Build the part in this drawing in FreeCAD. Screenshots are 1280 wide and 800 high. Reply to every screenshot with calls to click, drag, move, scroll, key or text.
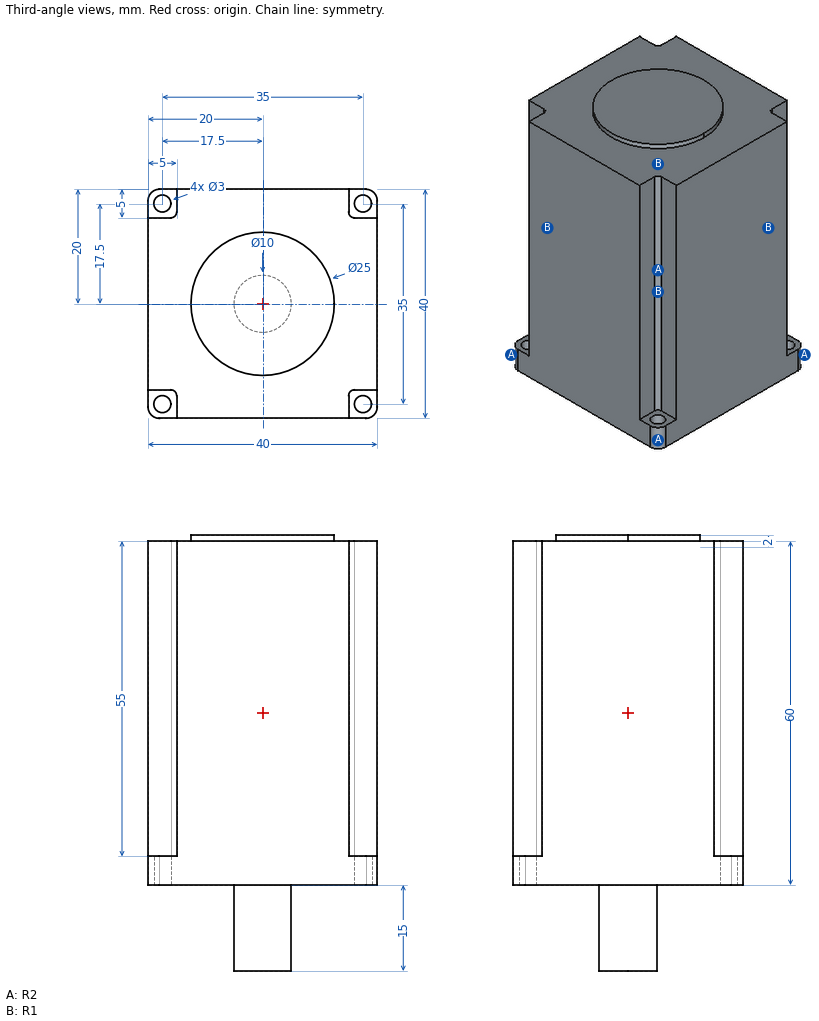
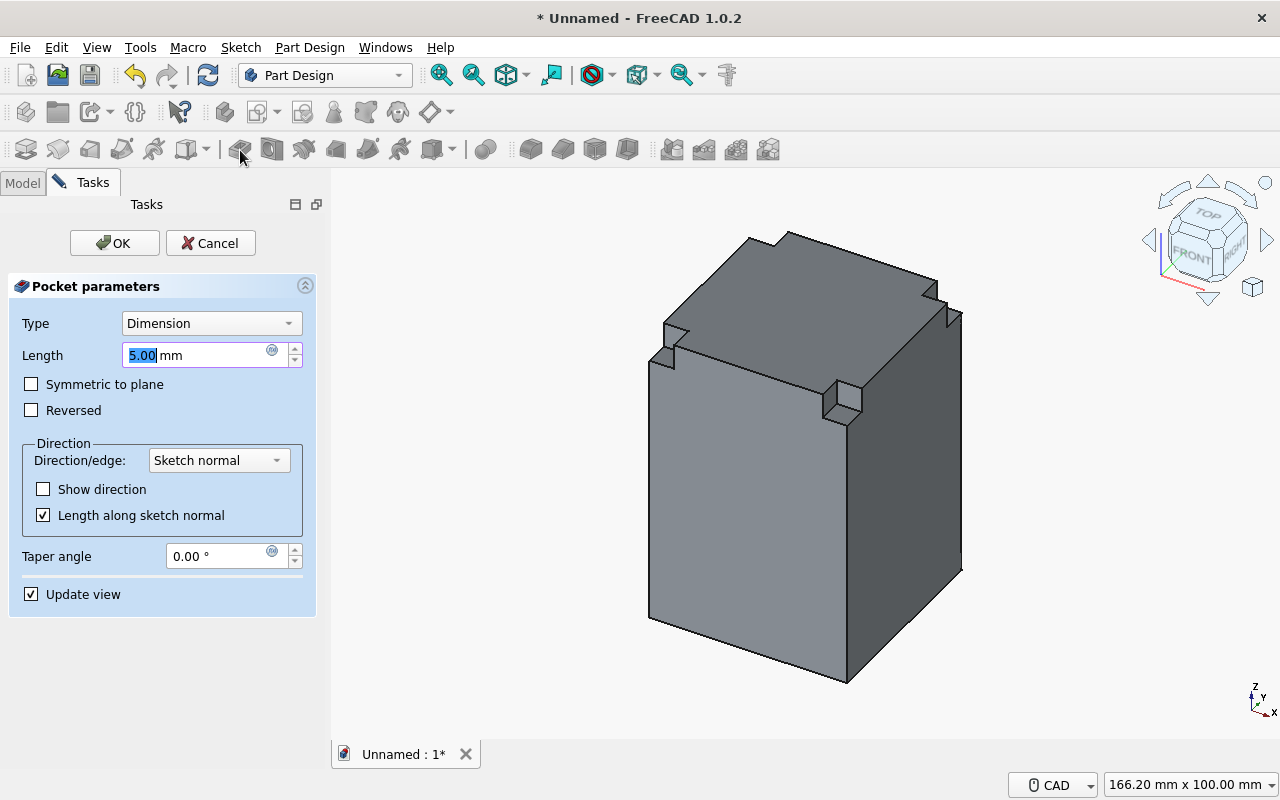
text(55)
key(Tab)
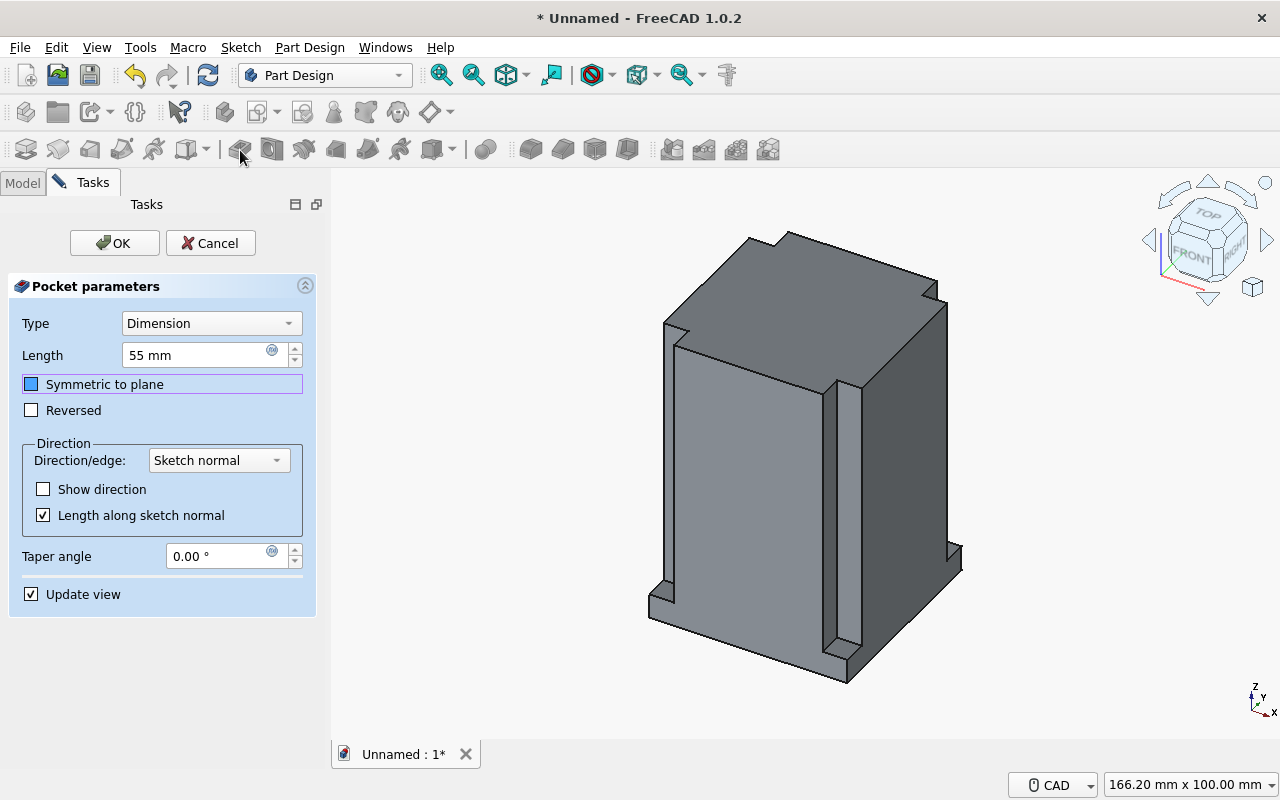
click(115, 243)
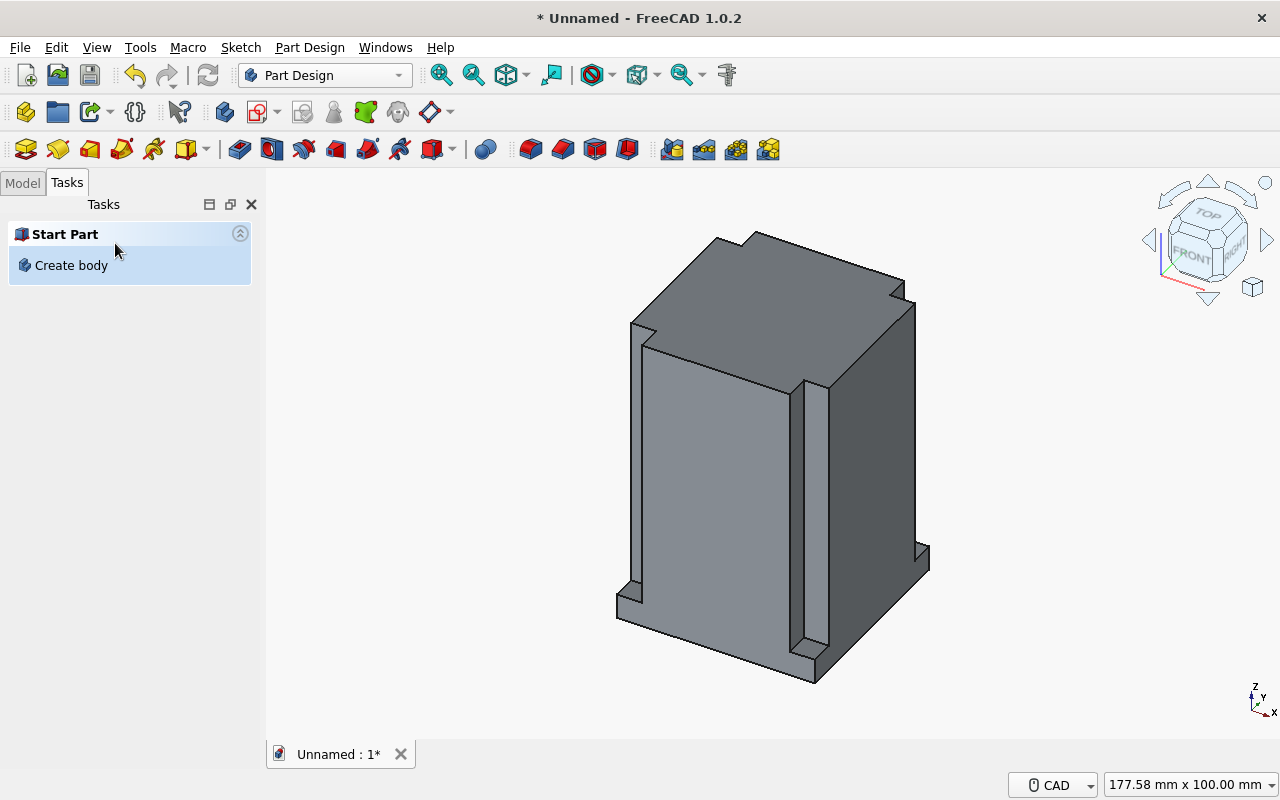
click(633, 589)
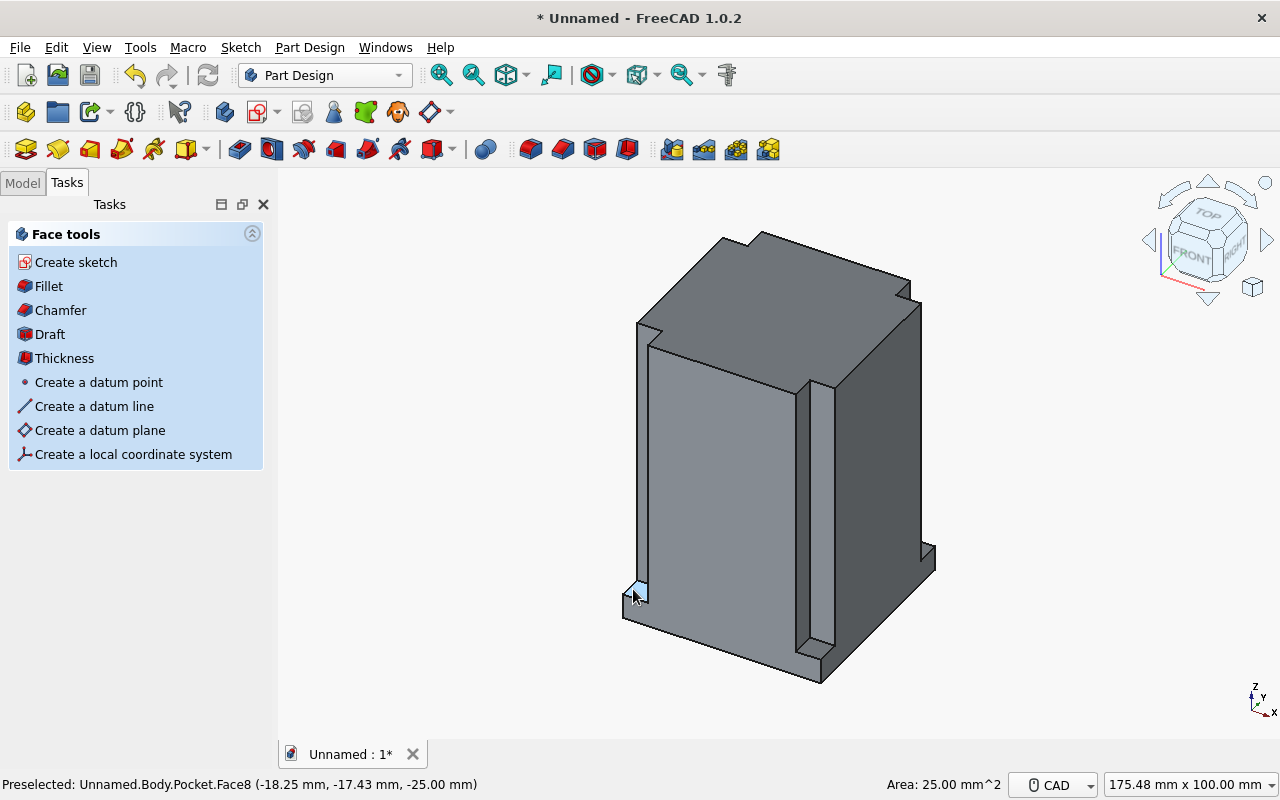
click(258, 112)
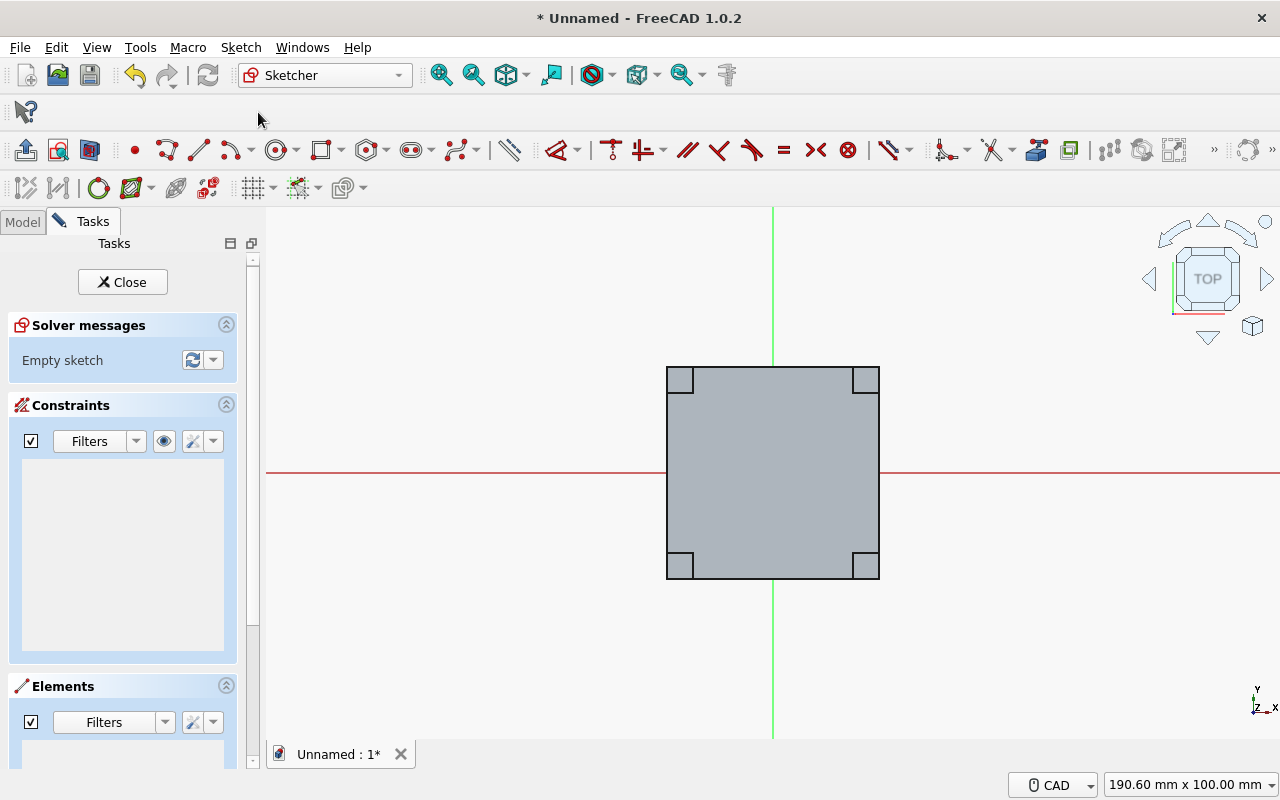
scroll(856, 473, up, 3)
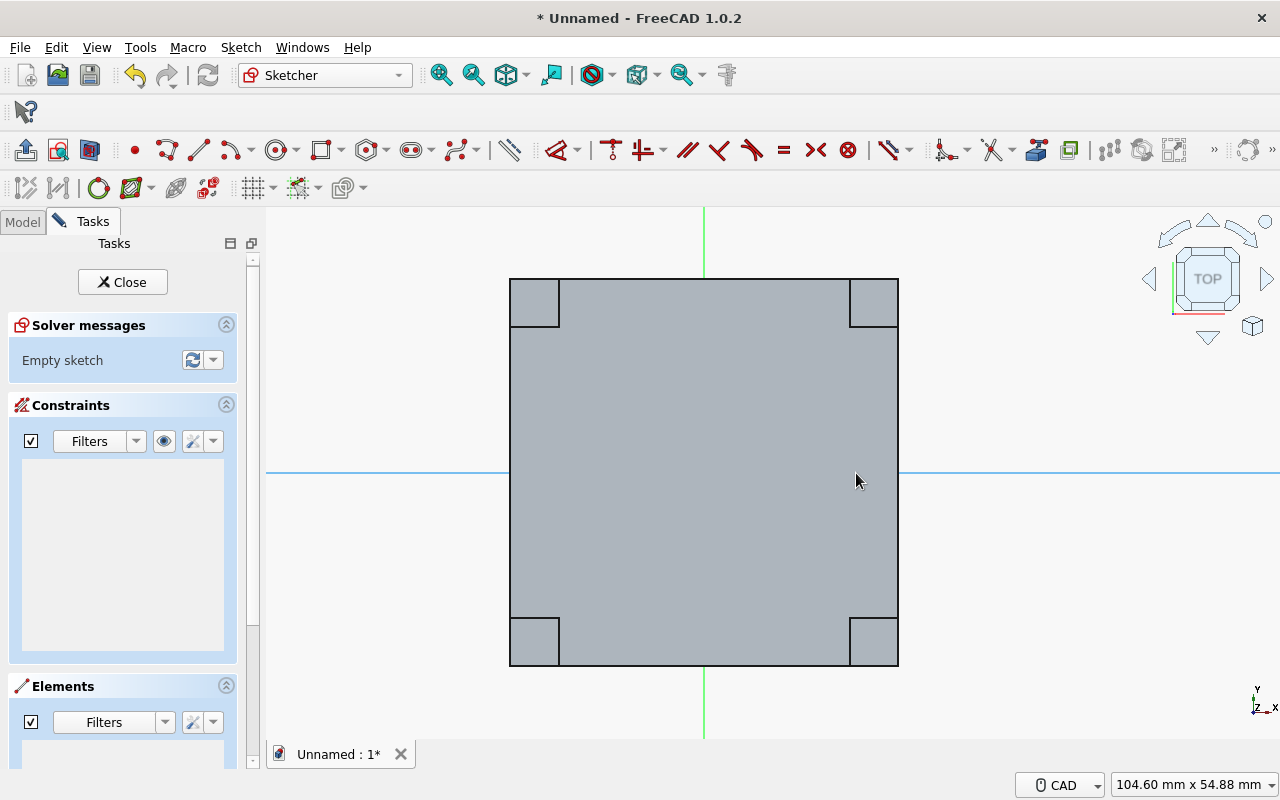
click(276, 150)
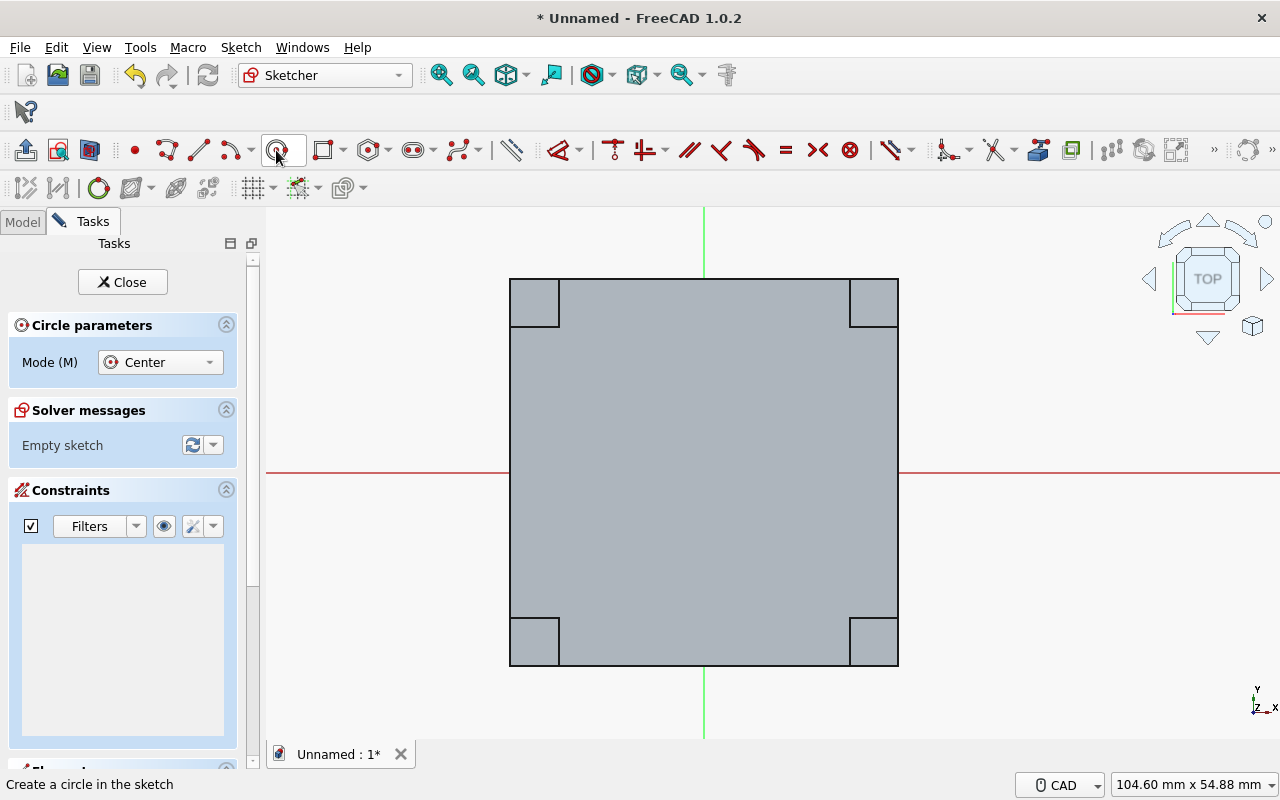
scroll(535, 303, up, 3)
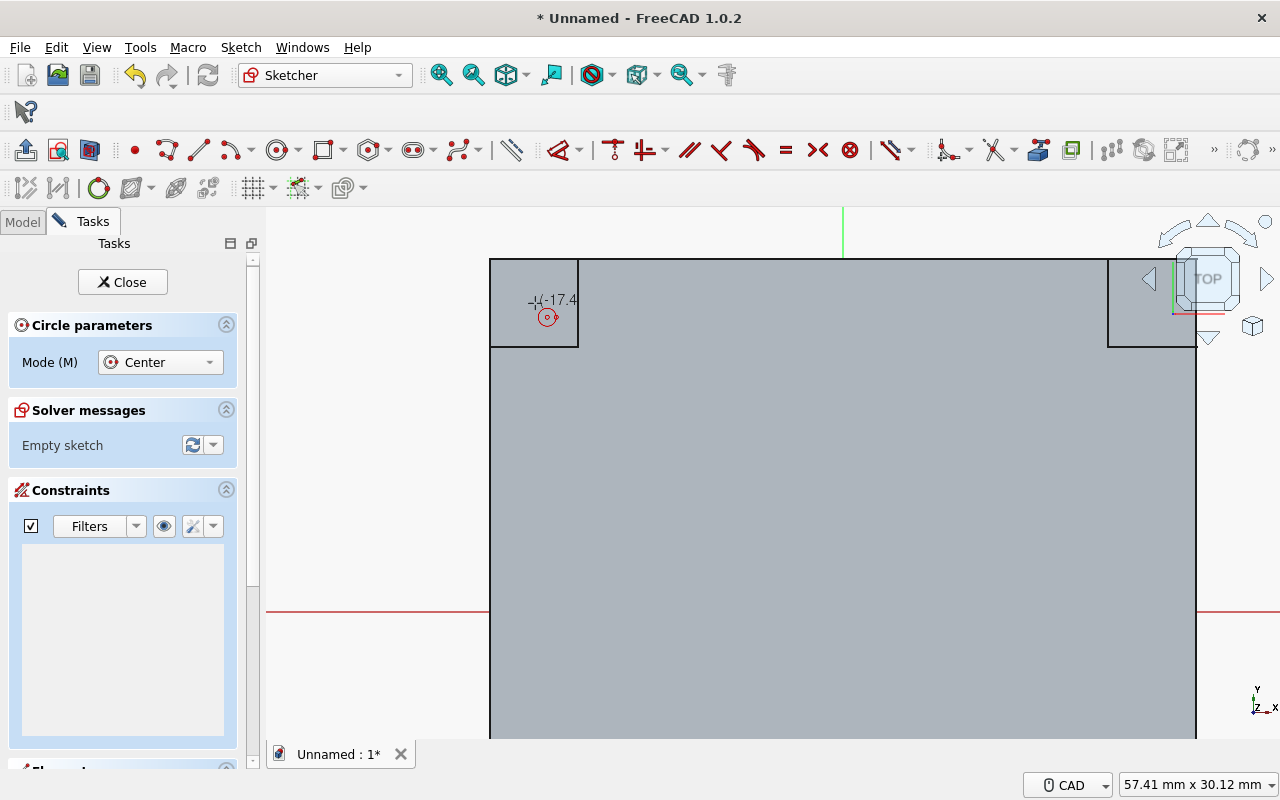
click(534, 303)
click(553, 284)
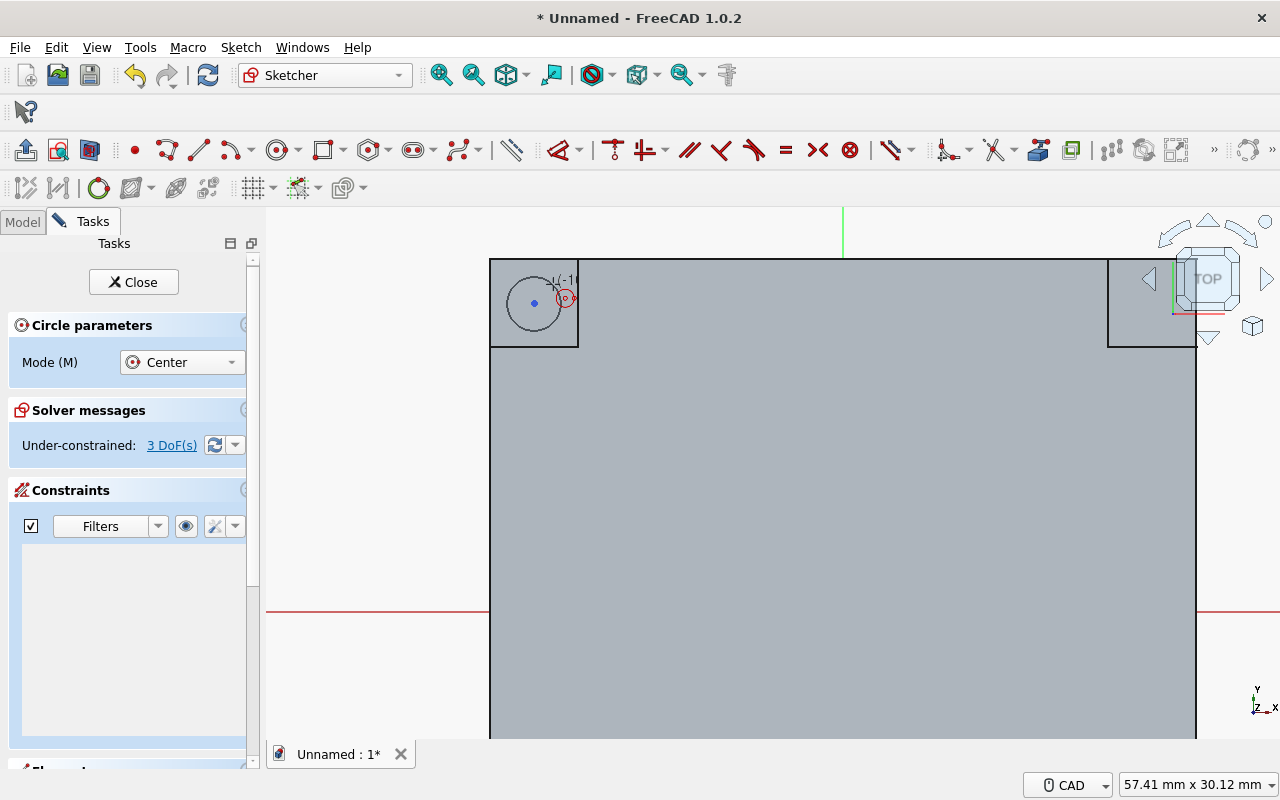
scroll(536, 304, down, 3)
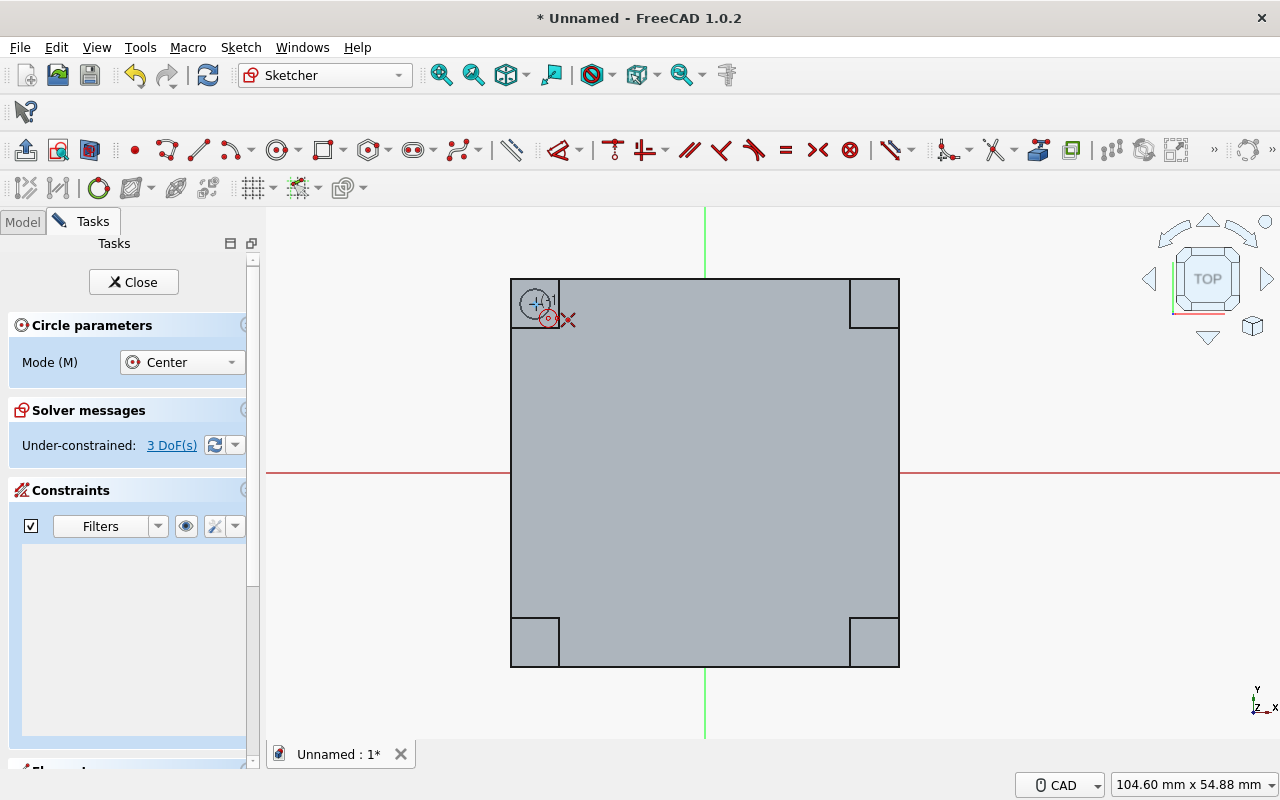
scroll(874, 303, up, 3)